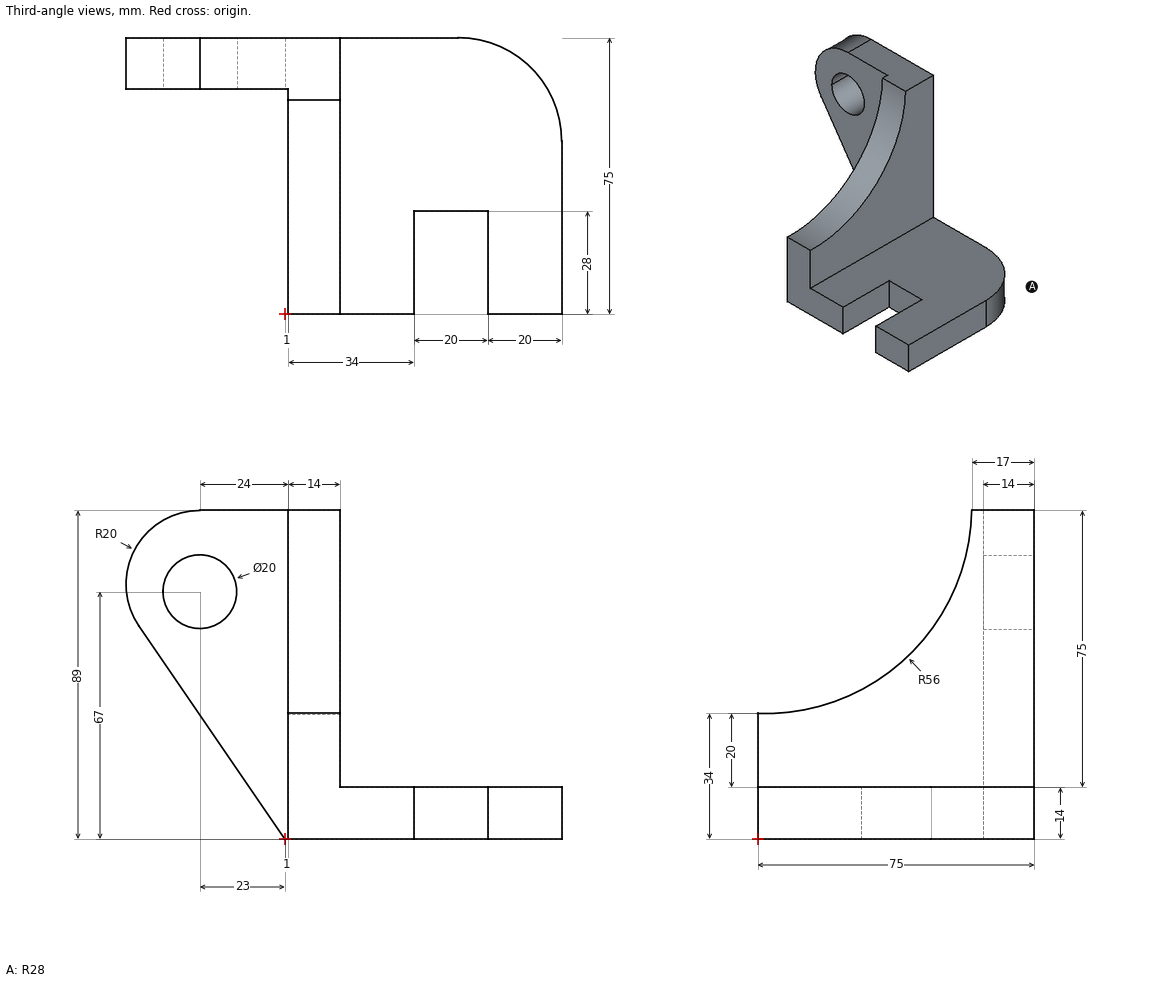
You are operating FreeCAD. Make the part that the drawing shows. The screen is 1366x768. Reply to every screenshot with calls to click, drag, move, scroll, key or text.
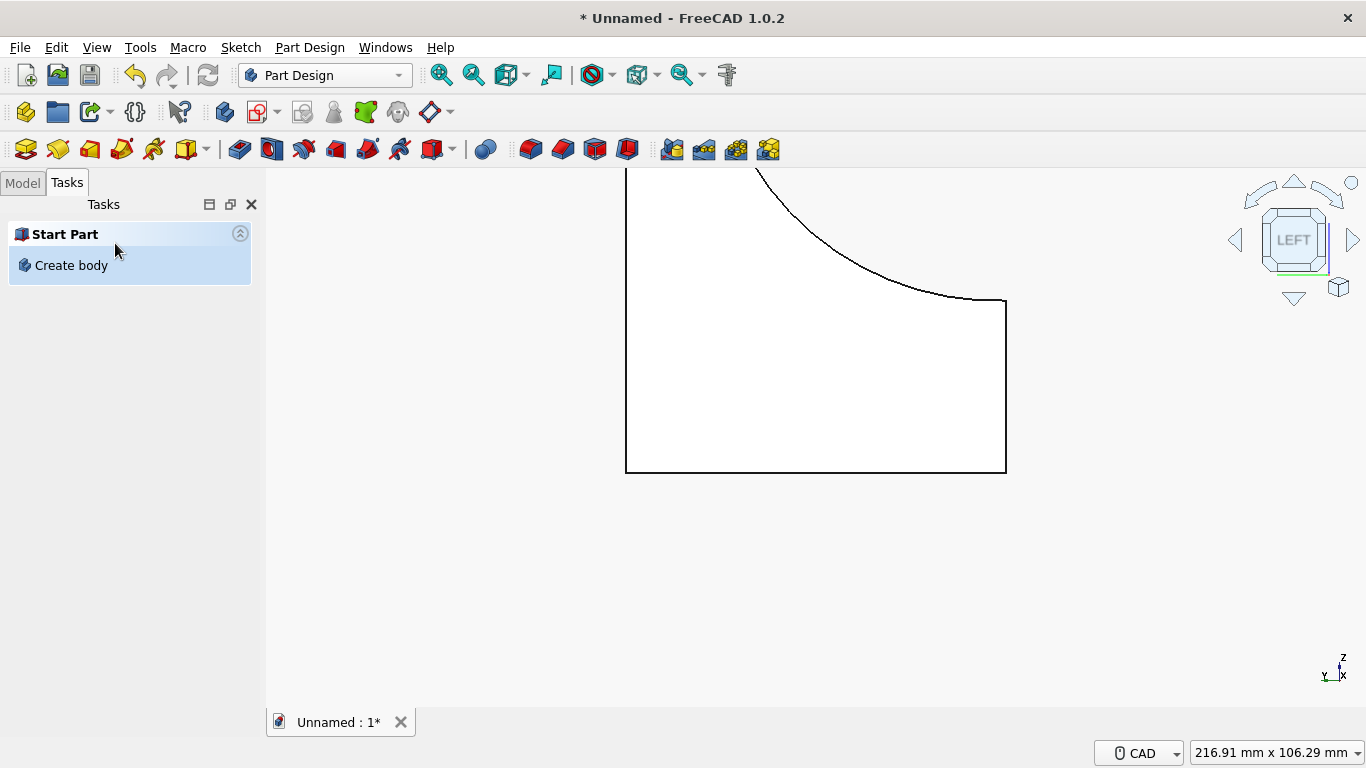
click(442, 76)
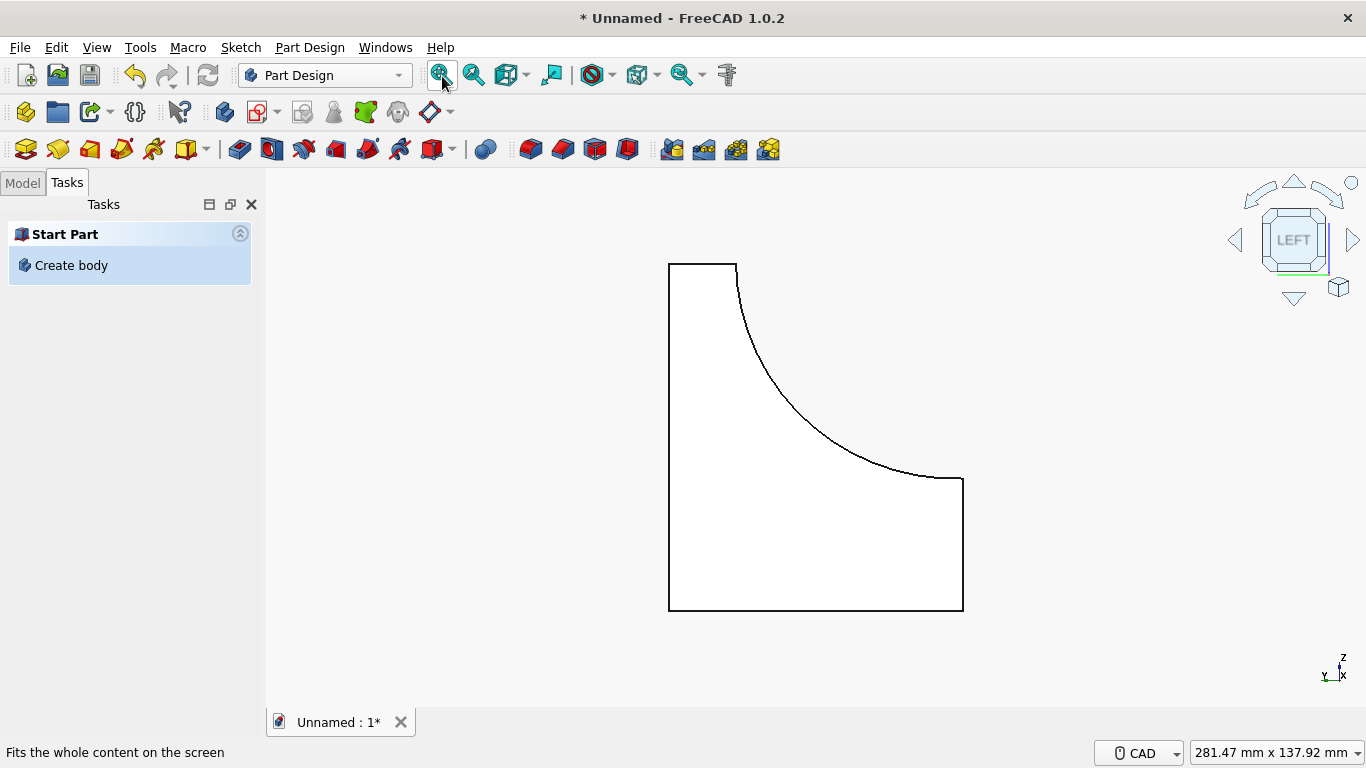
key(4)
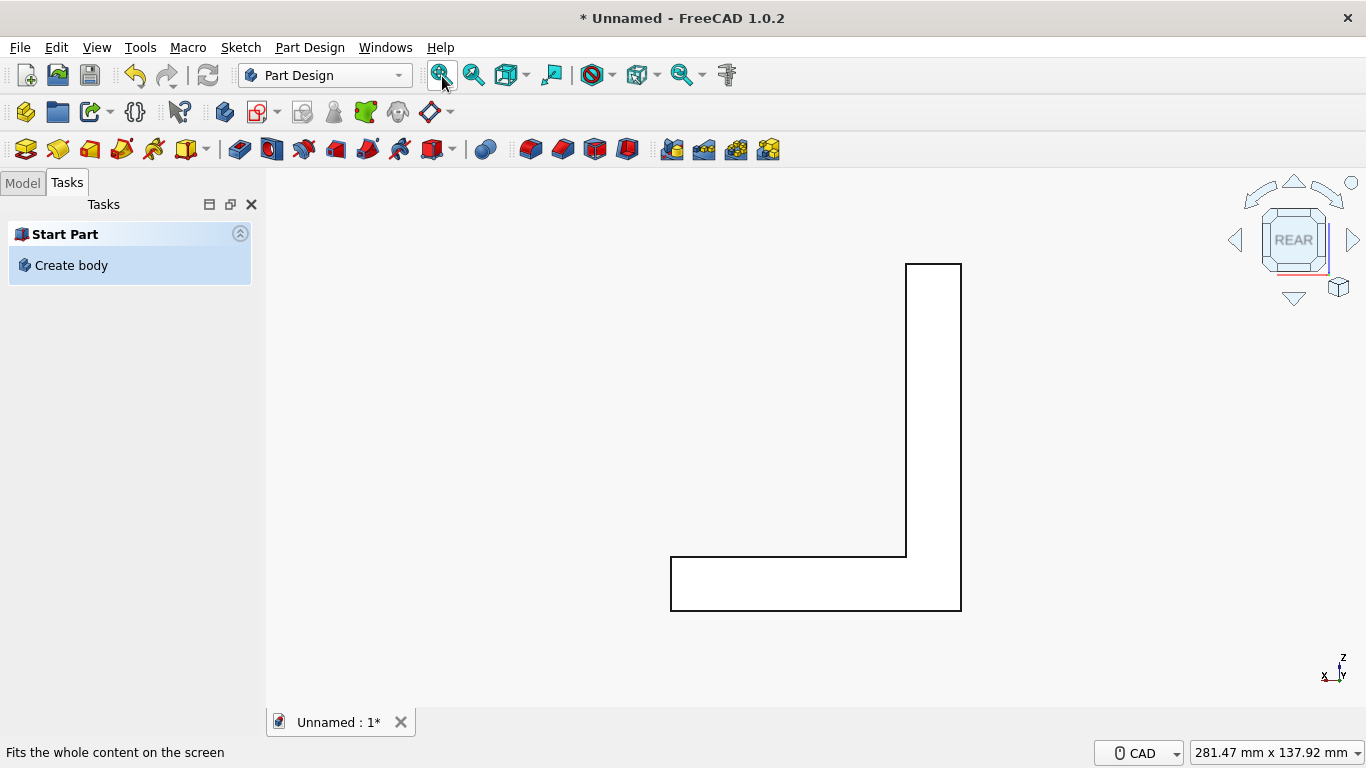
click(733, 586)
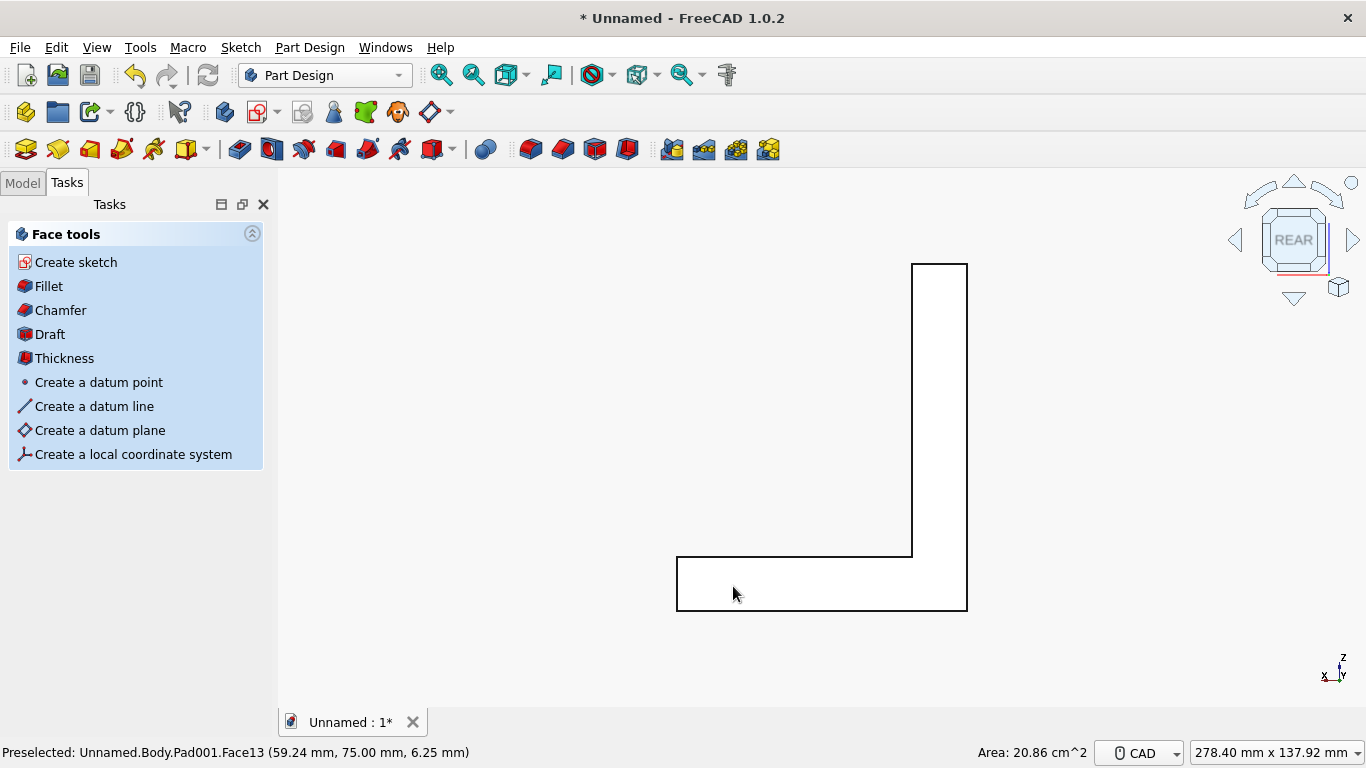
click(258, 112)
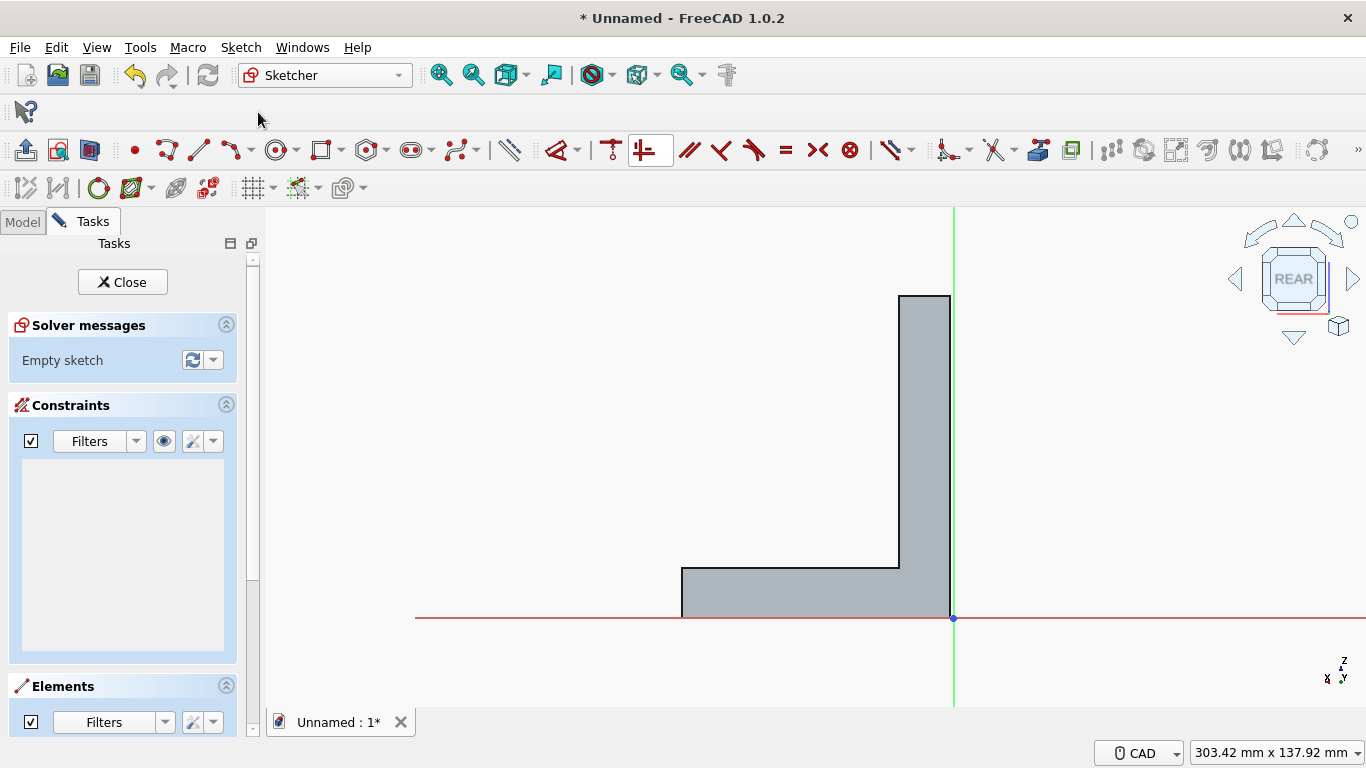
click(168, 150)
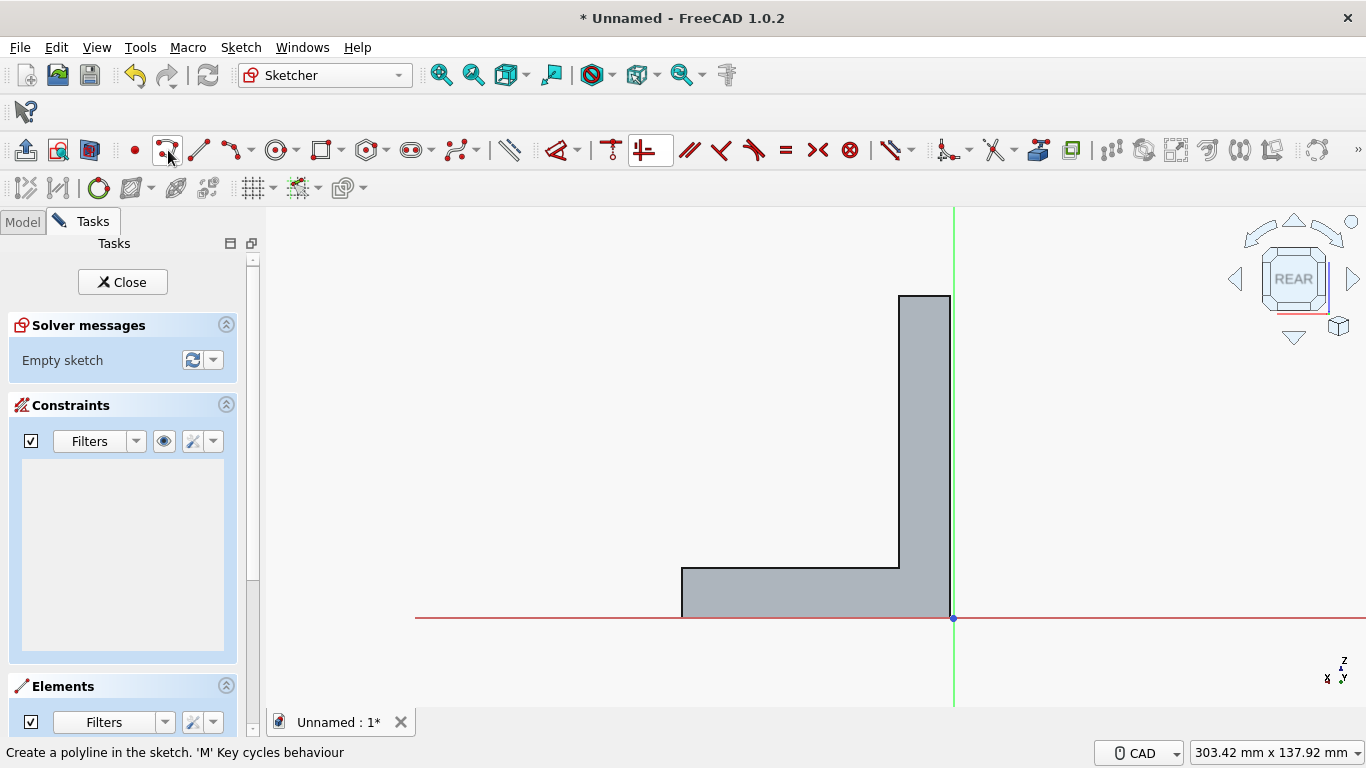
click(1037, 296)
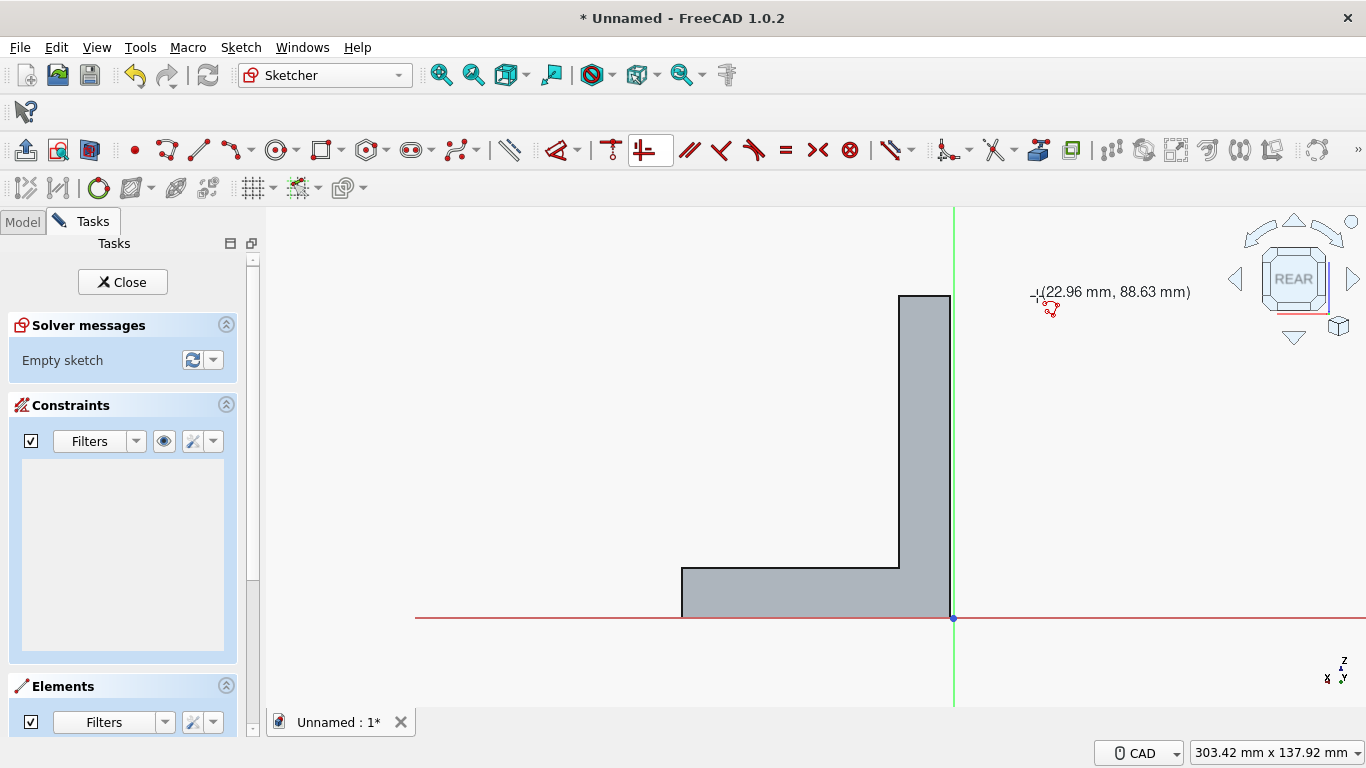
scroll(950, 296, up, 8)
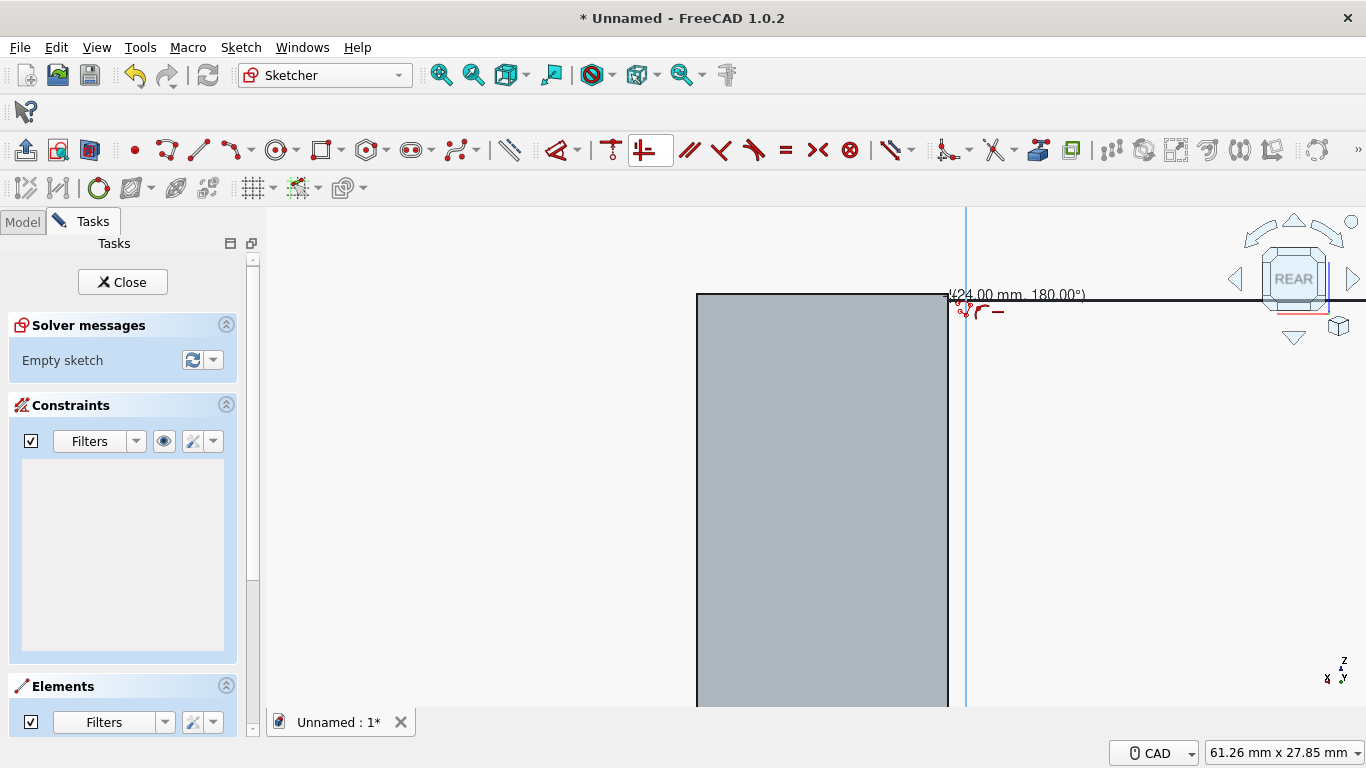
click(948, 295)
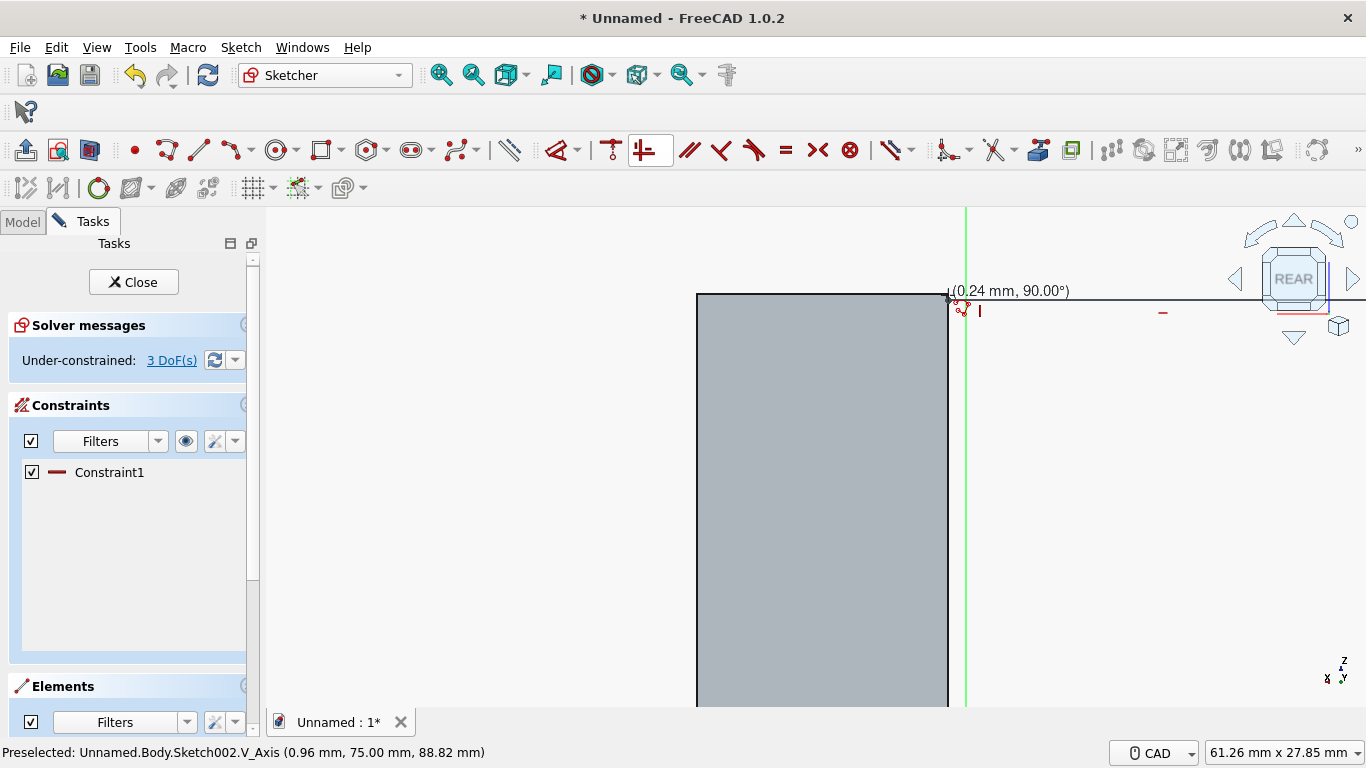
scroll(602, 296, down, 8)